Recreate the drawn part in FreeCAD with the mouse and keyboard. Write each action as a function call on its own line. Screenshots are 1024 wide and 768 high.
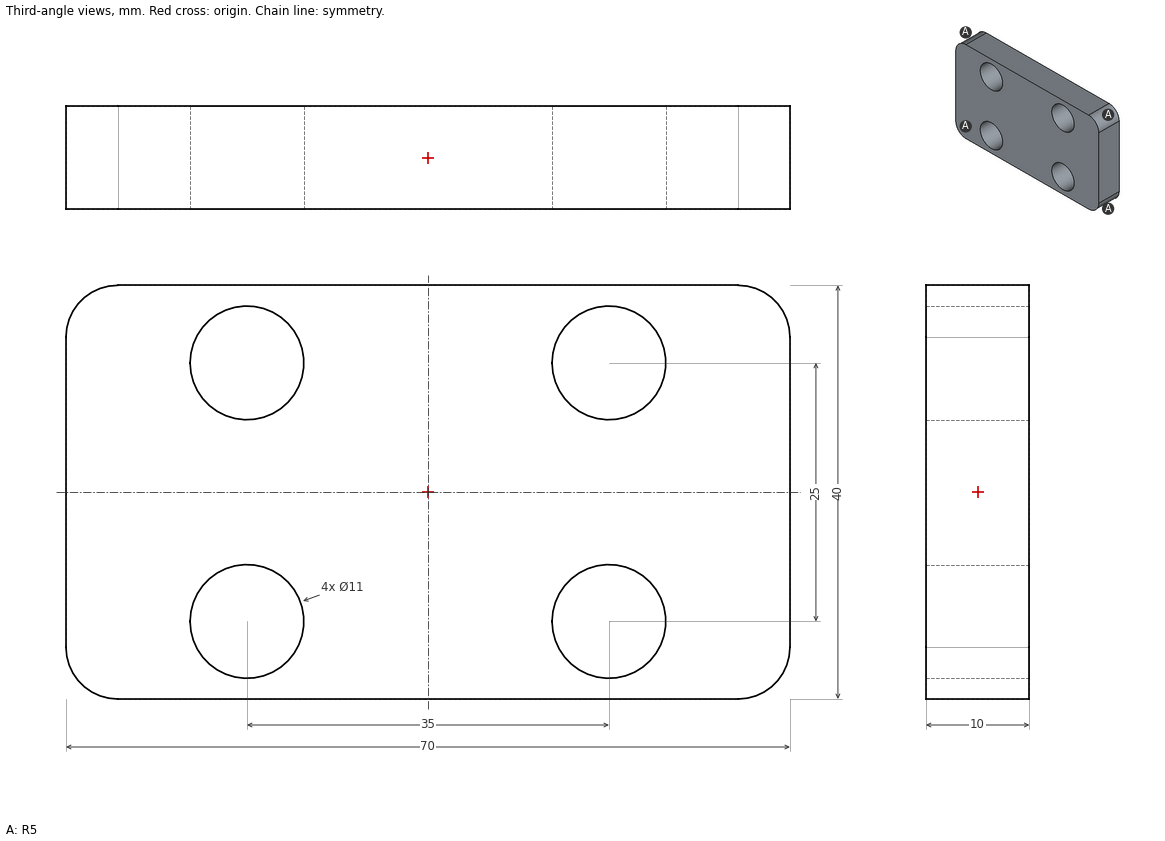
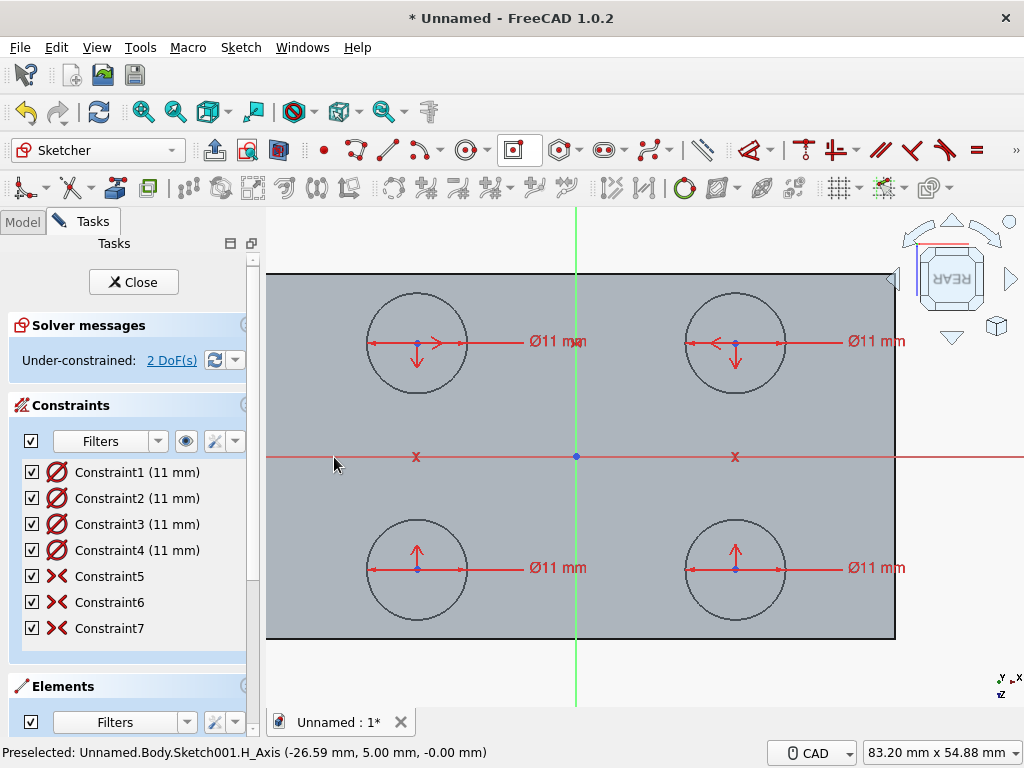
click(417, 343)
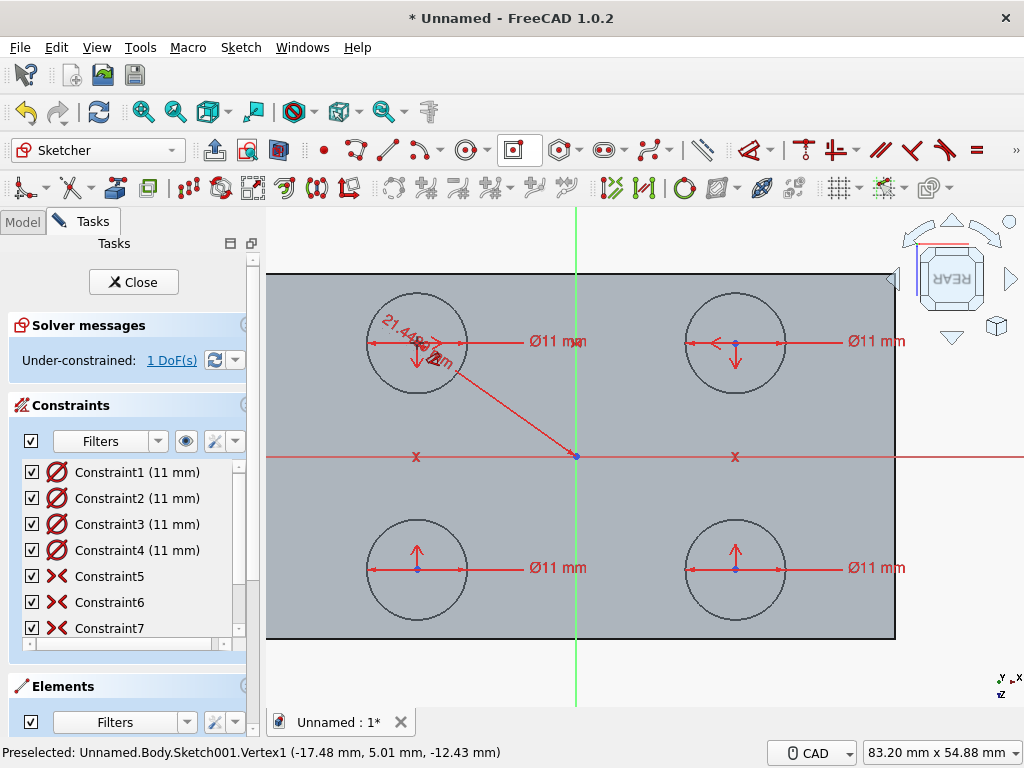
click(736, 343)
click(503, 309)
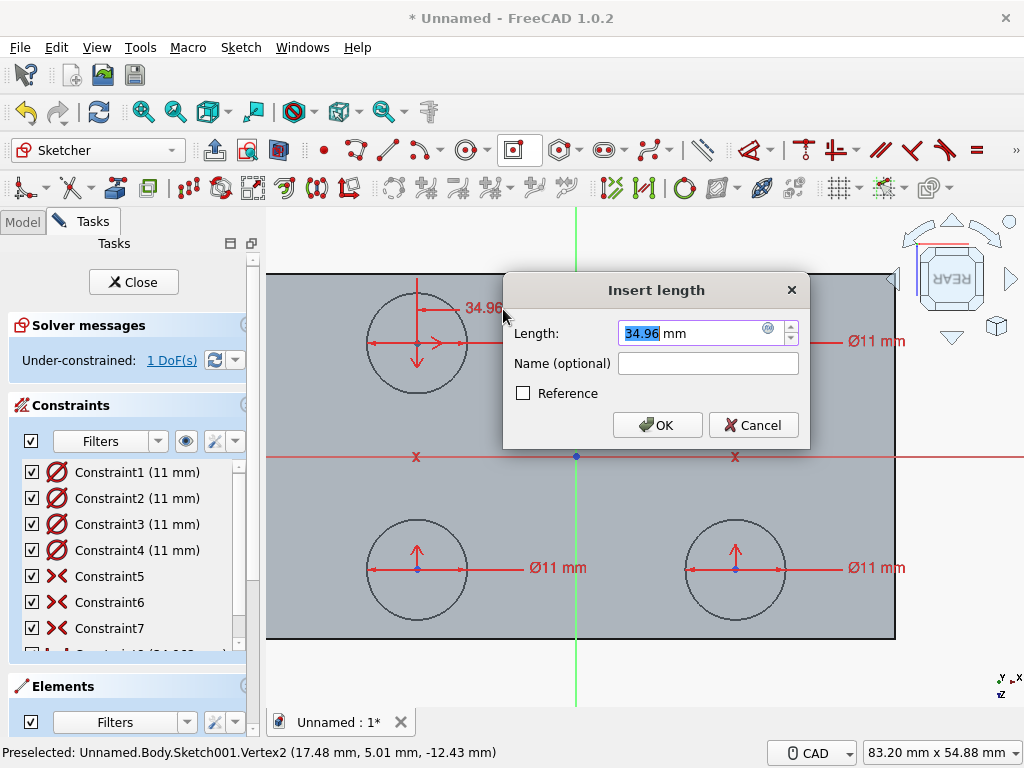
text(35)
key(Return)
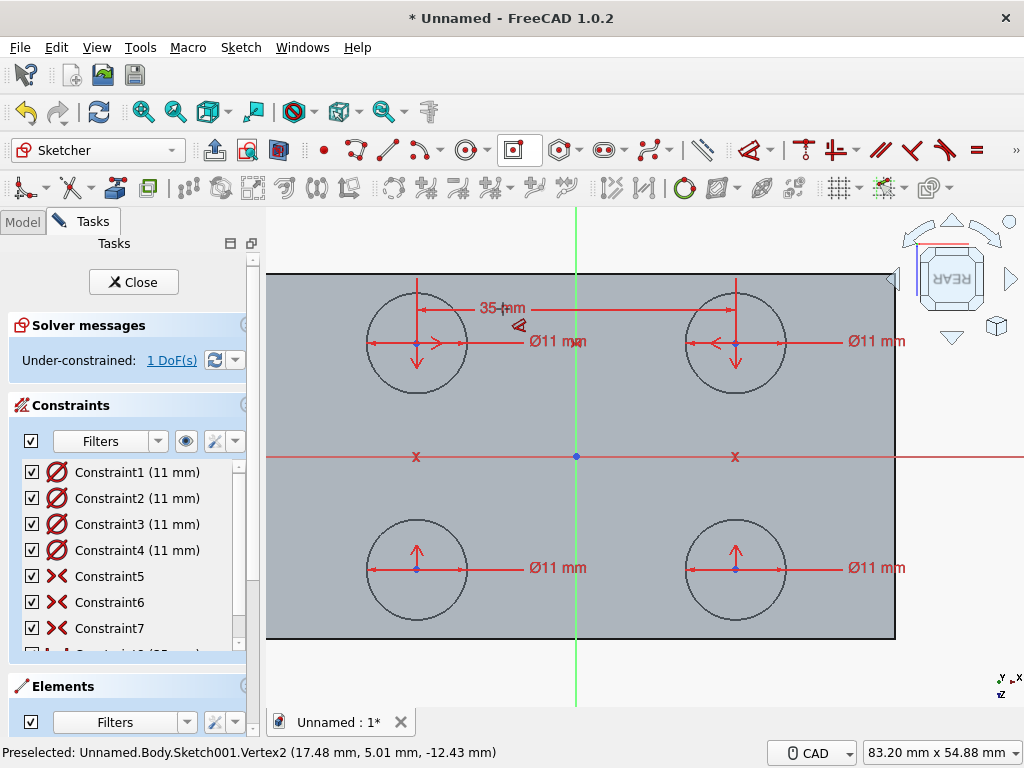
click(736, 343)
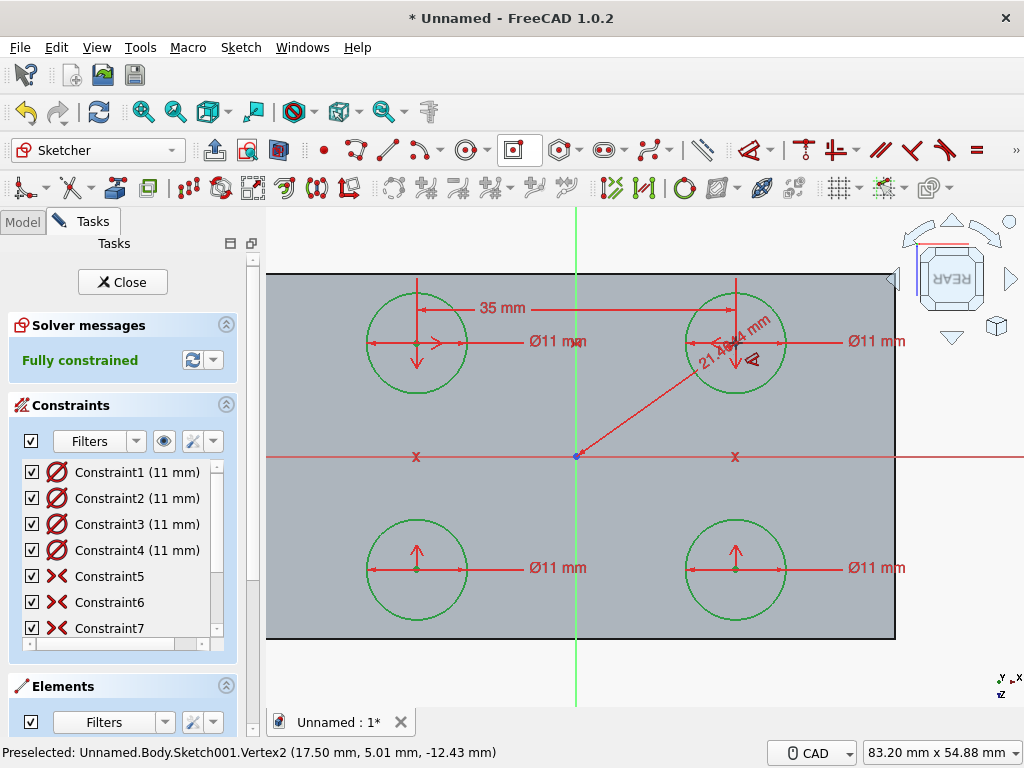
click(736, 570)
click(770, 405)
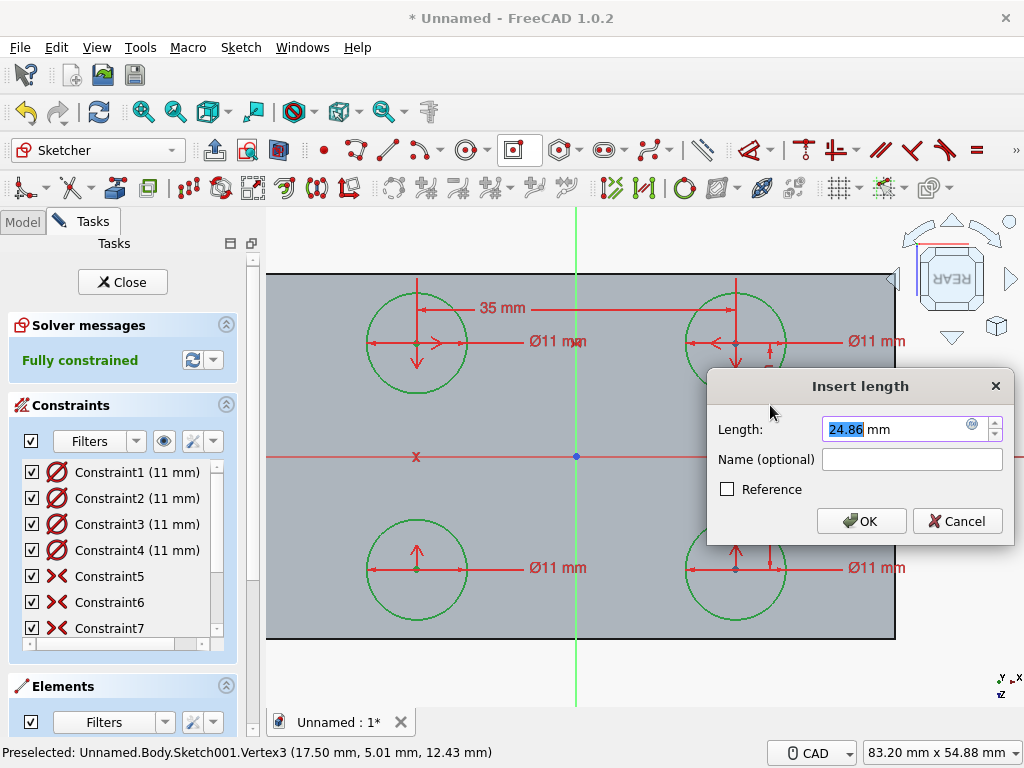
text(25)
key(Return)
key(Escape)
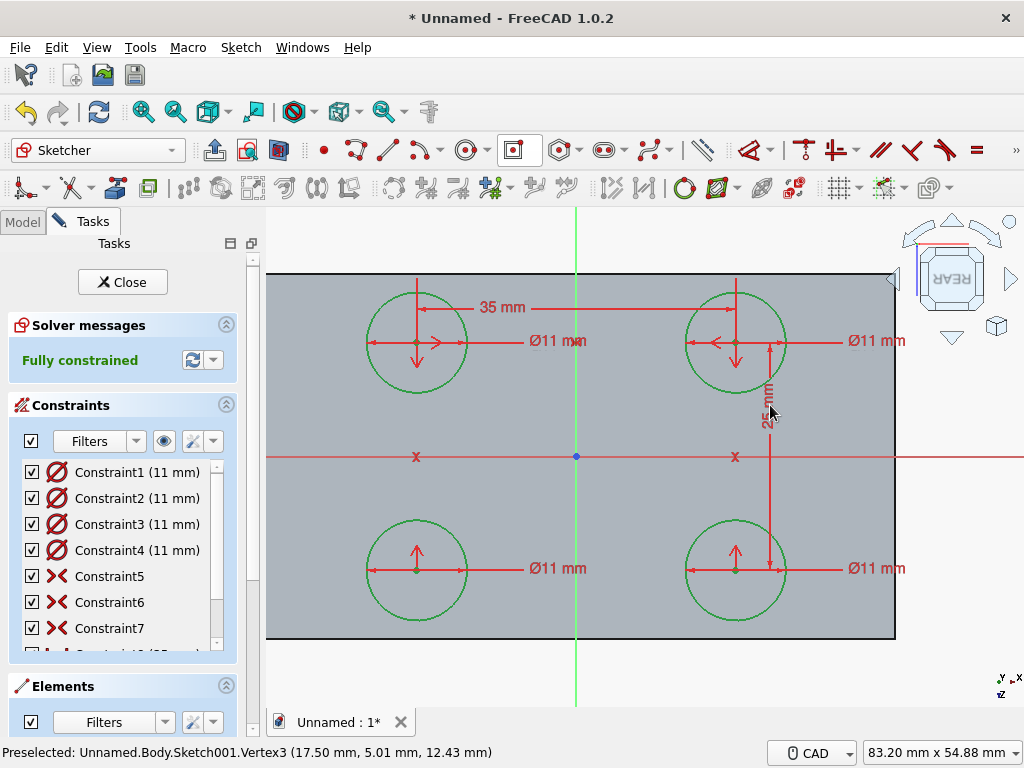
click(123, 282)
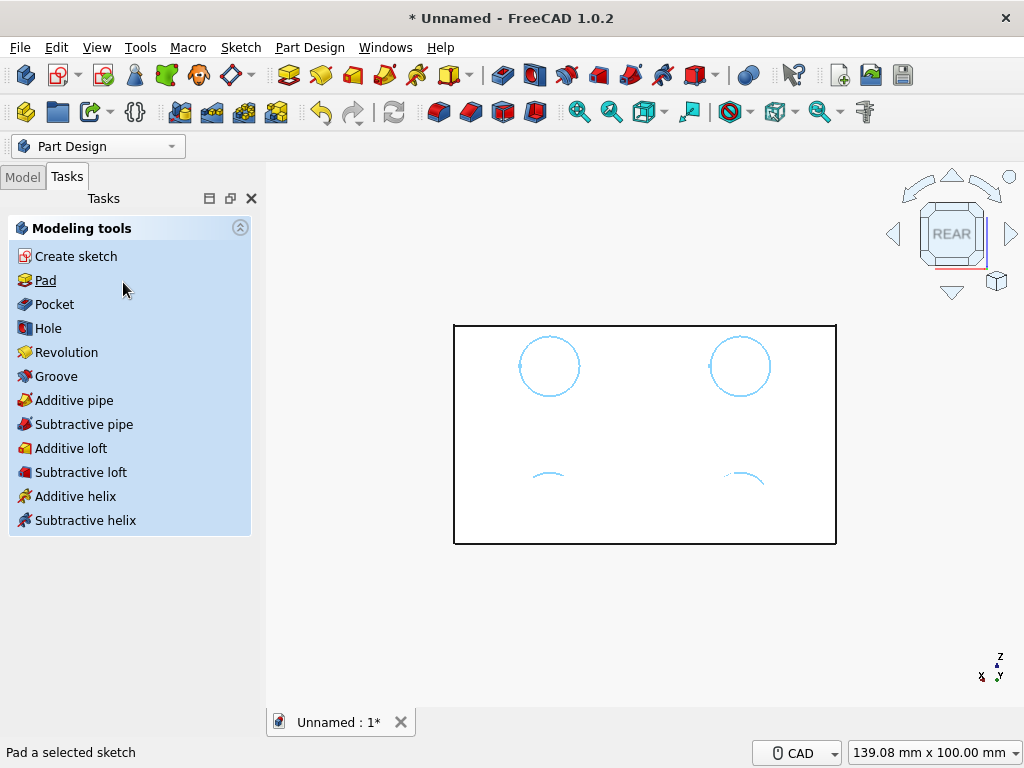
click(504, 76)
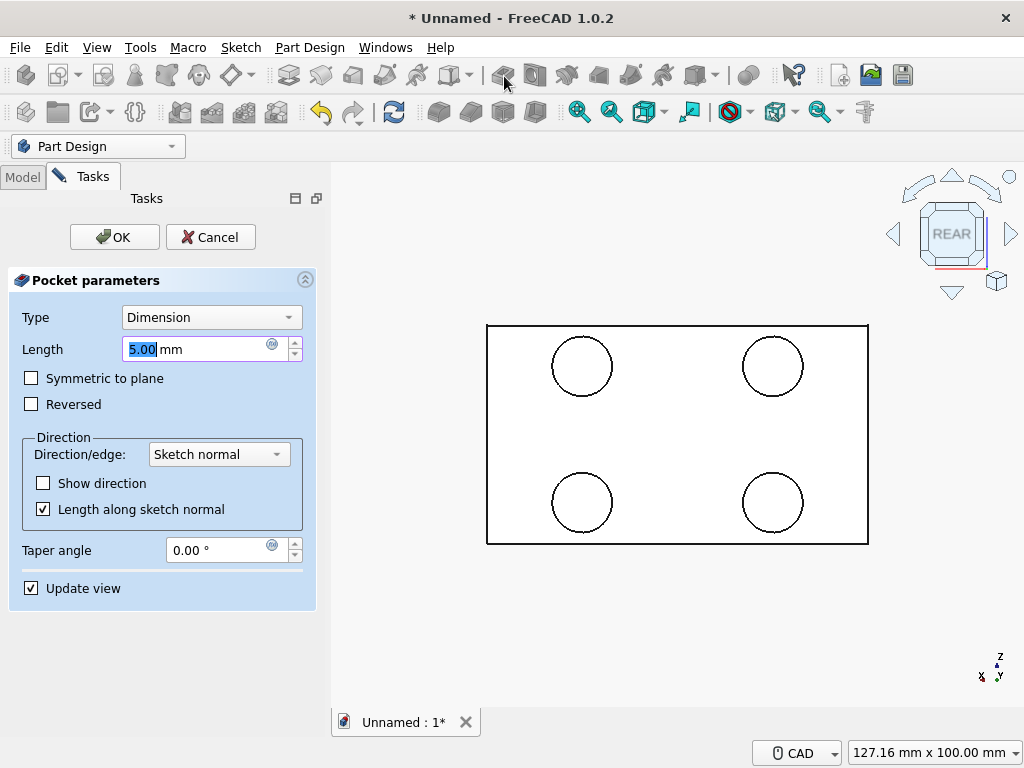
click(212, 318)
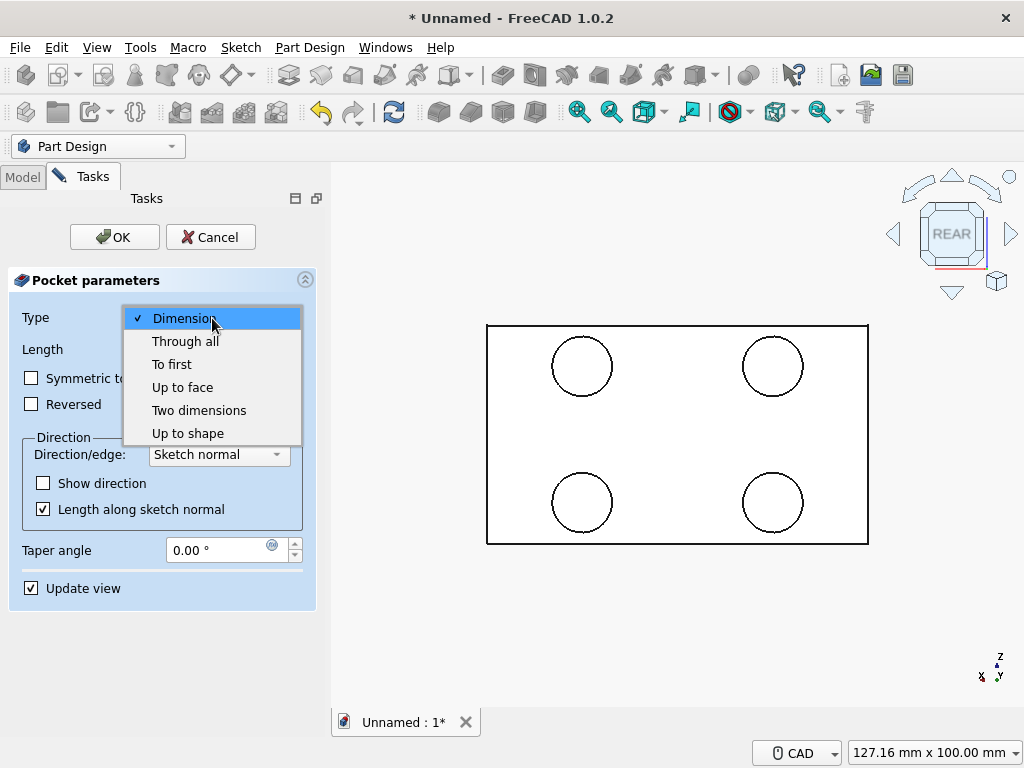
click(212, 342)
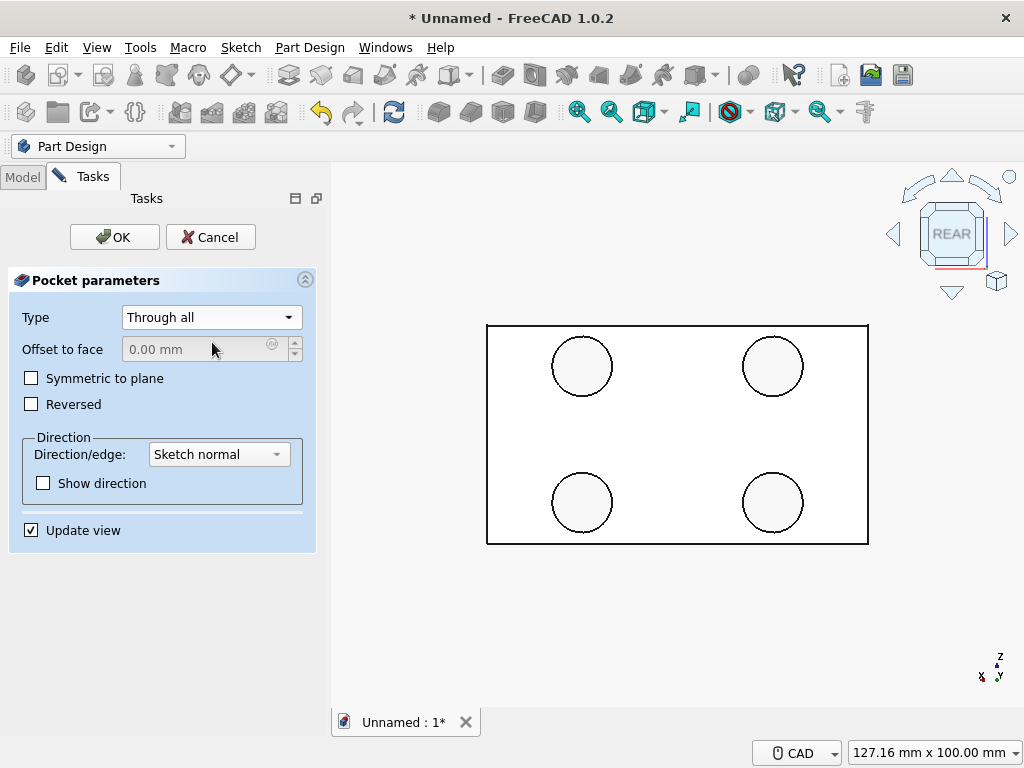
click(115, 237)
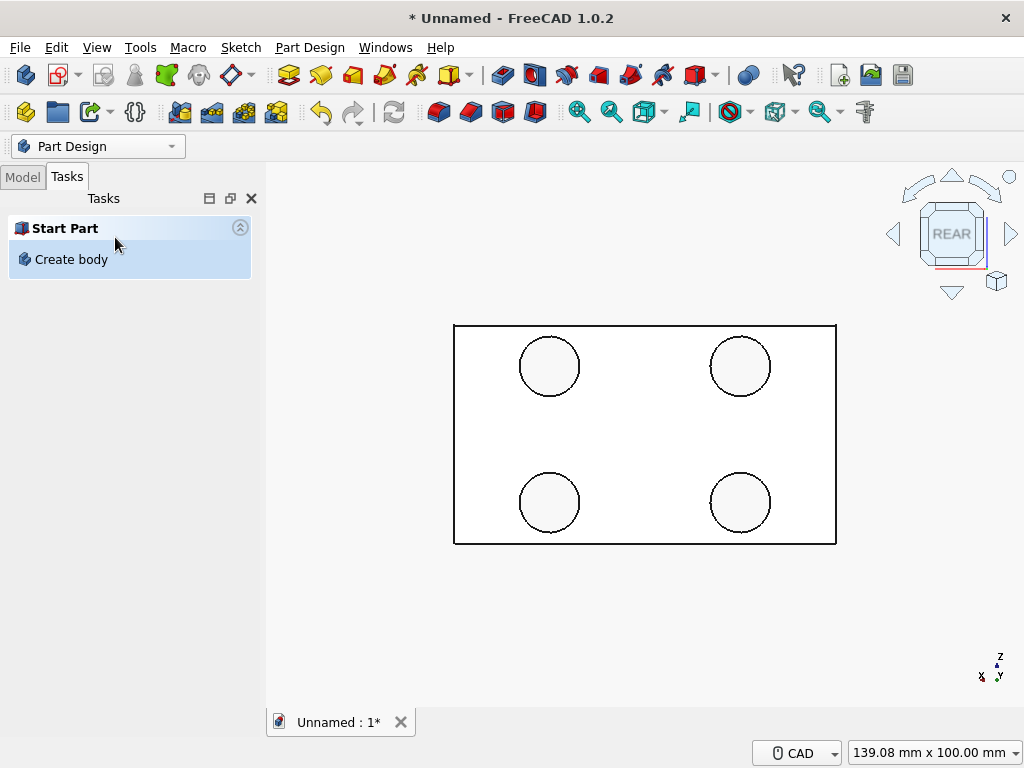
key(0)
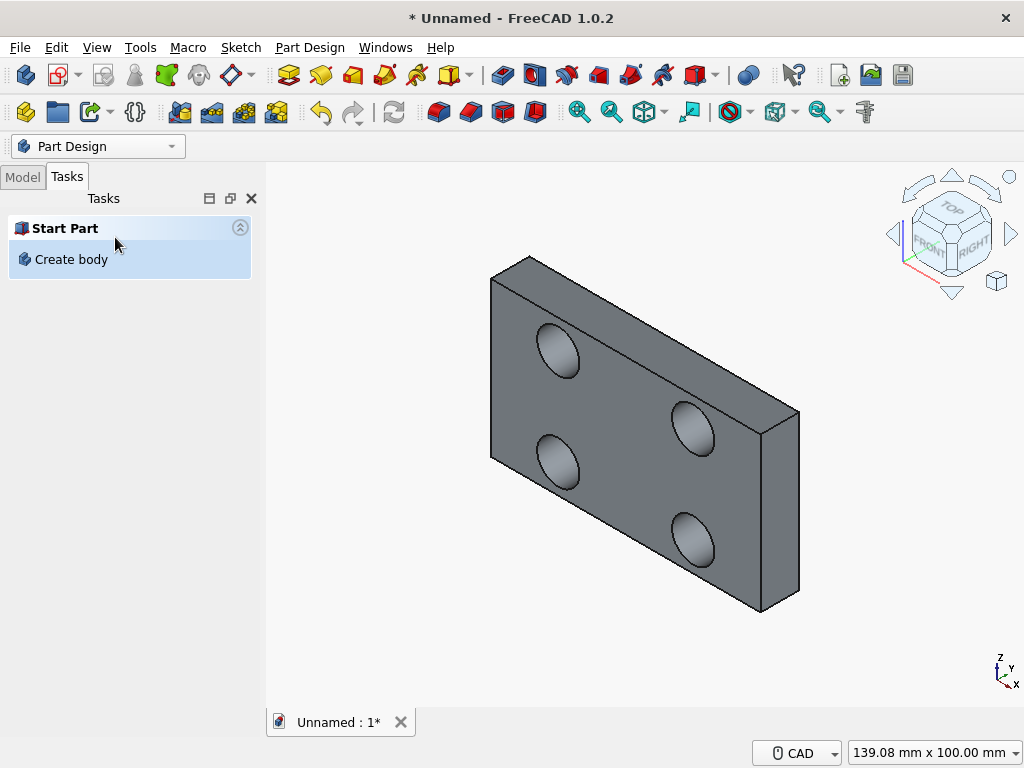
click(780, 422)